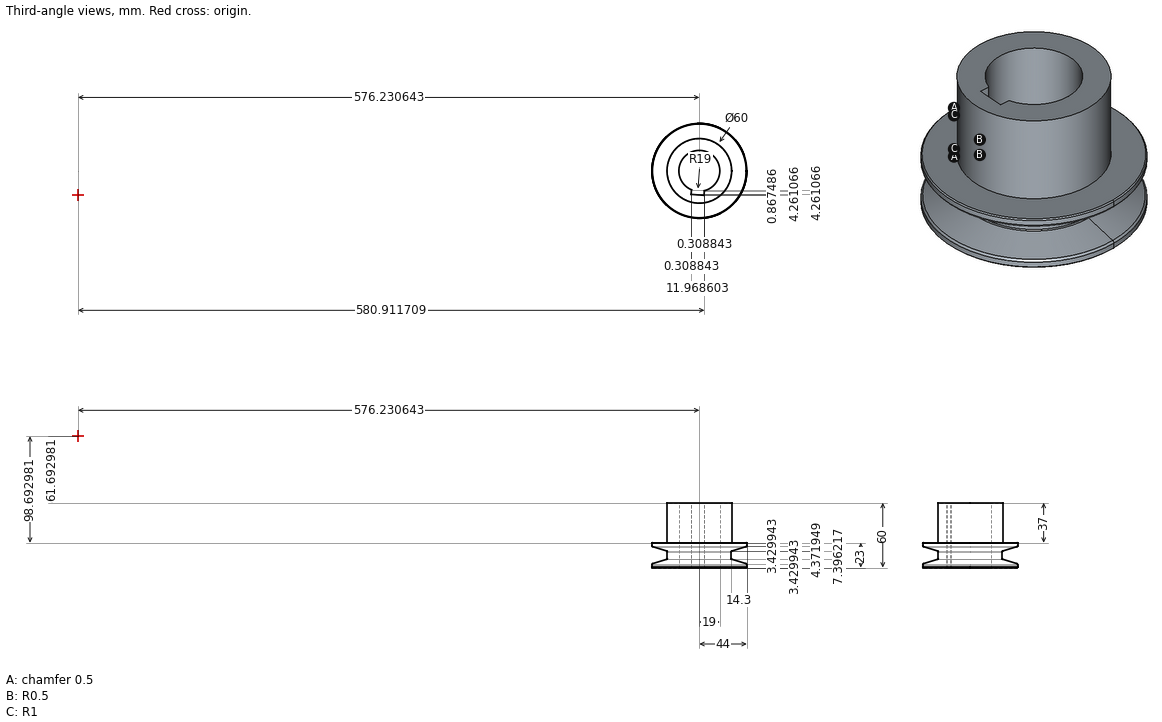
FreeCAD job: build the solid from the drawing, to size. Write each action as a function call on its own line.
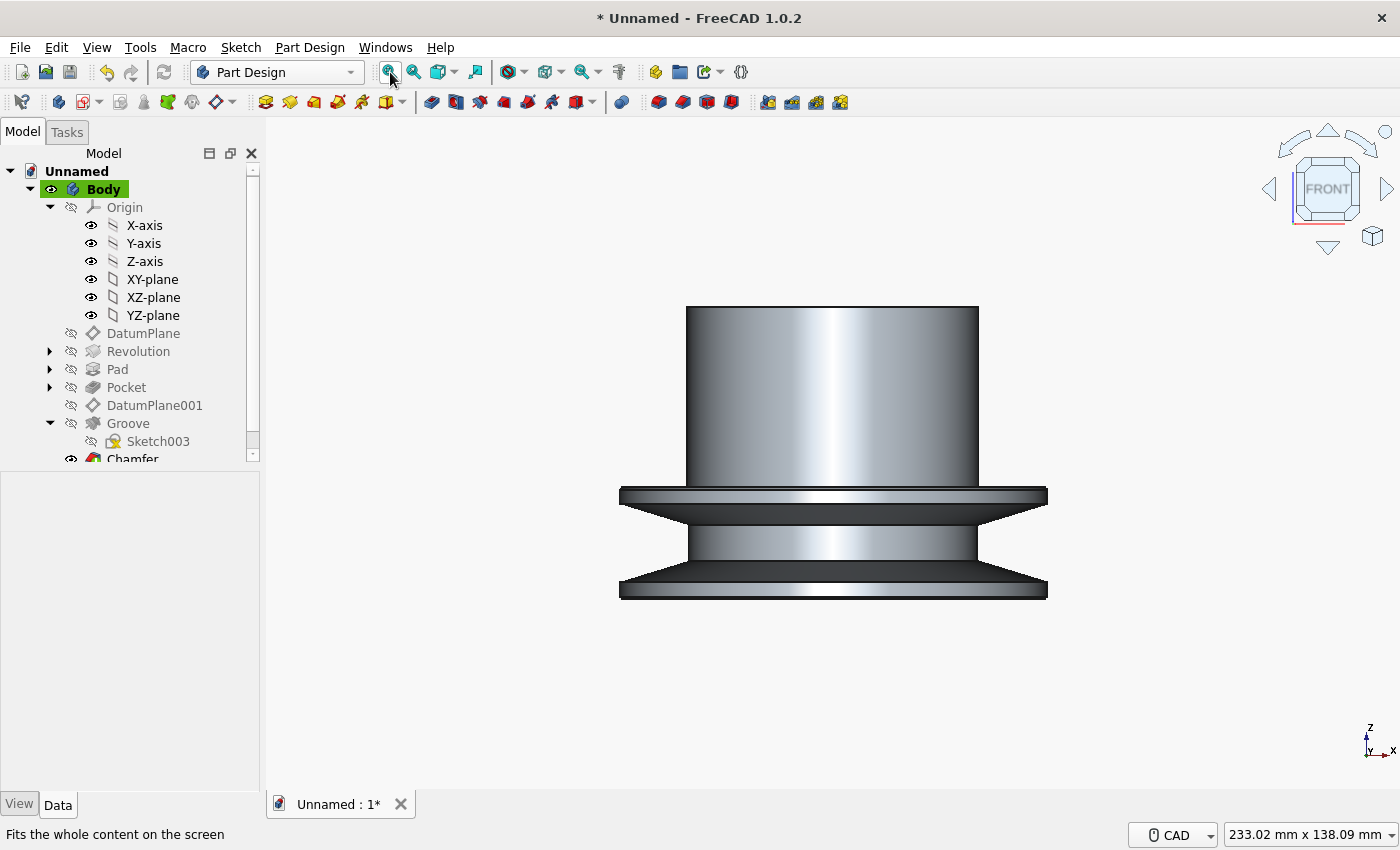
key(3)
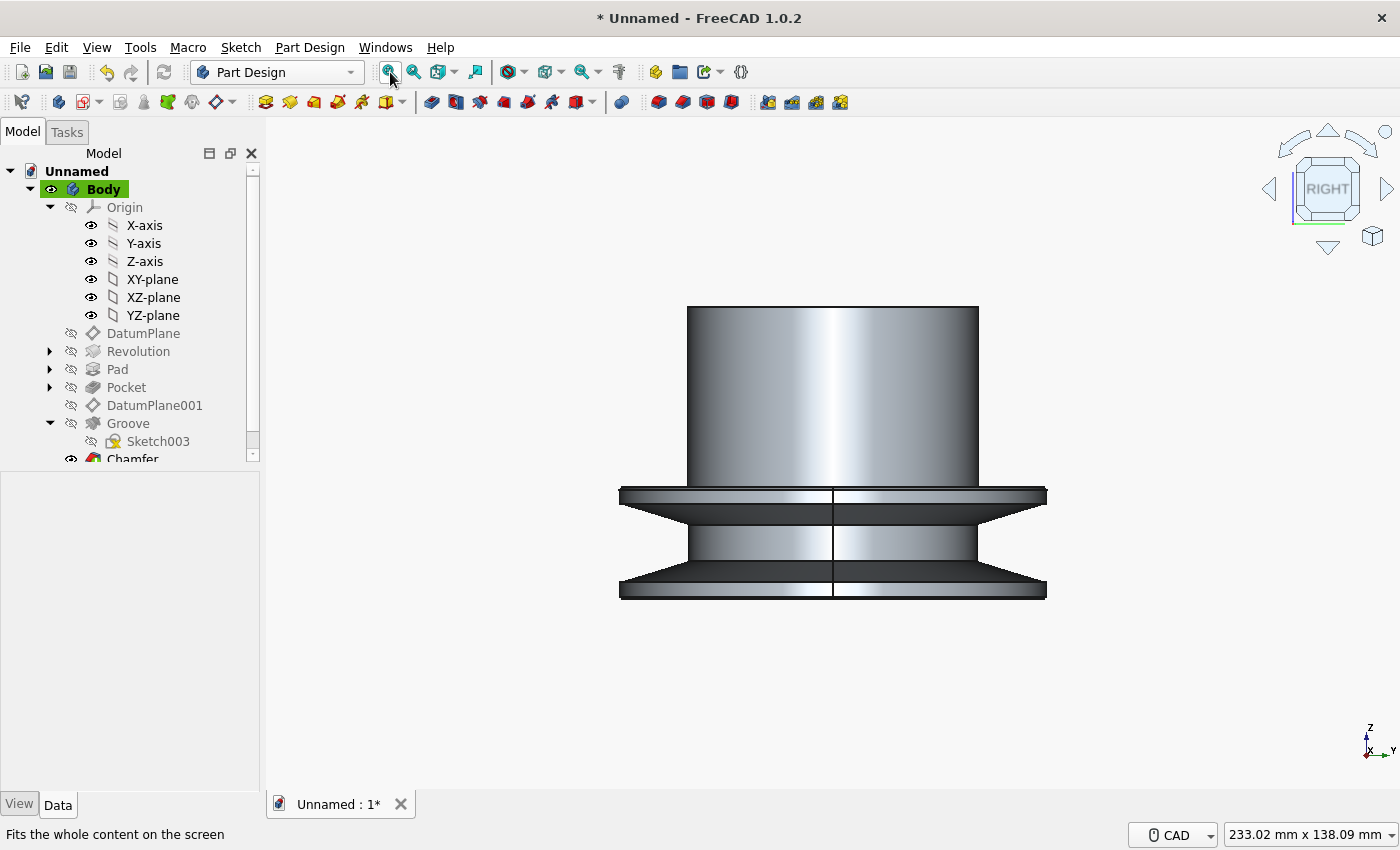
key(v)
key(f)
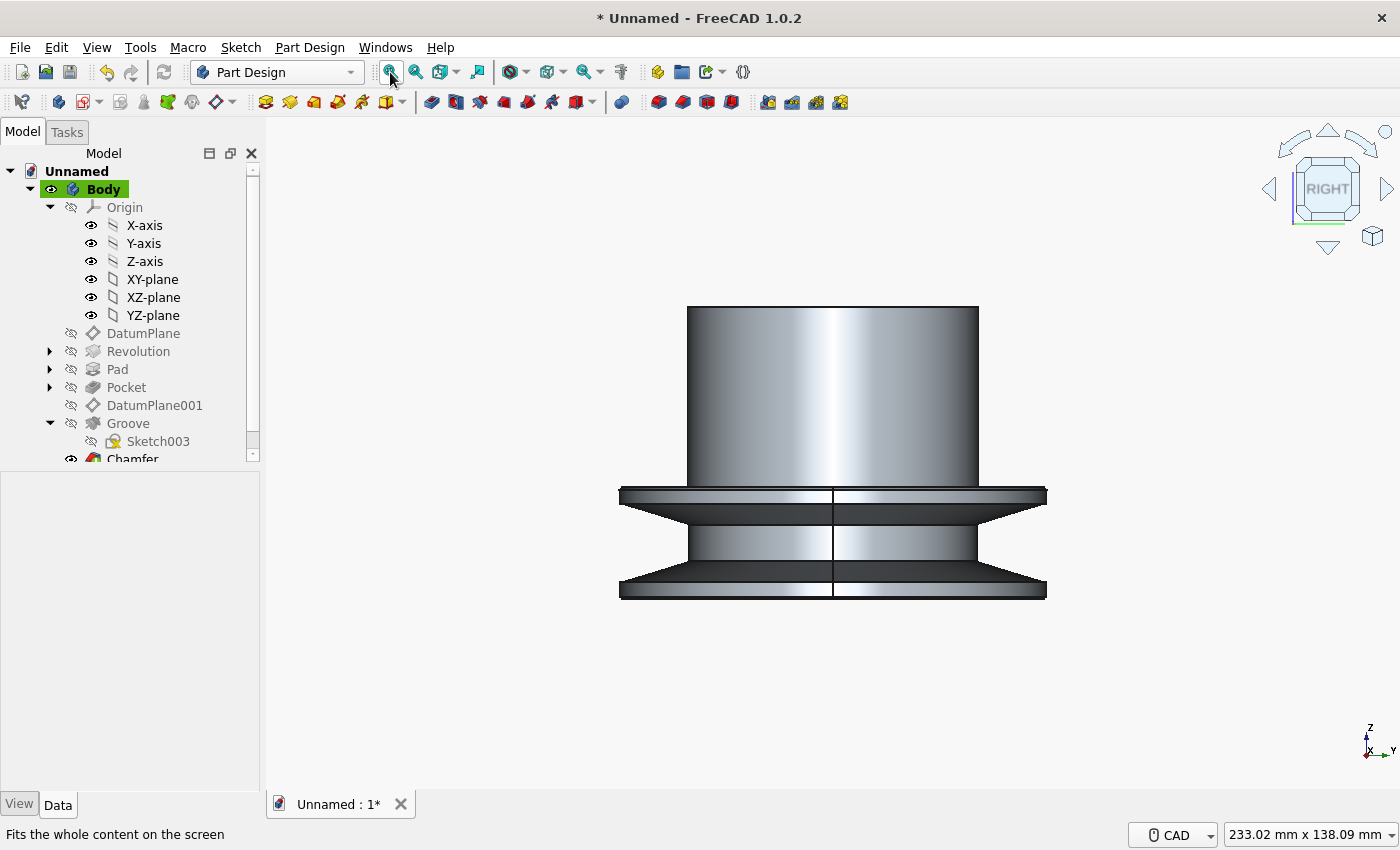
key(5)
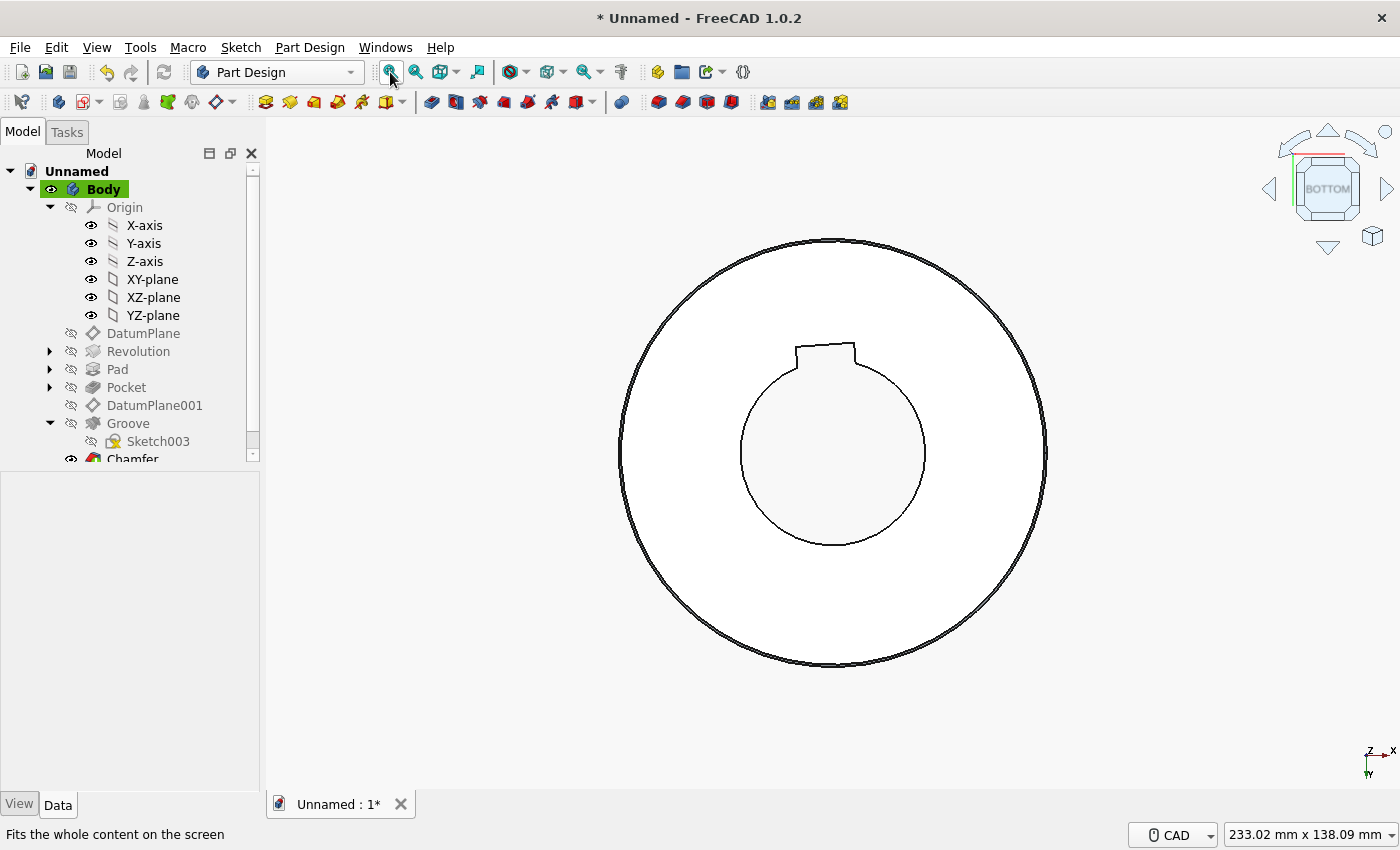
key(4)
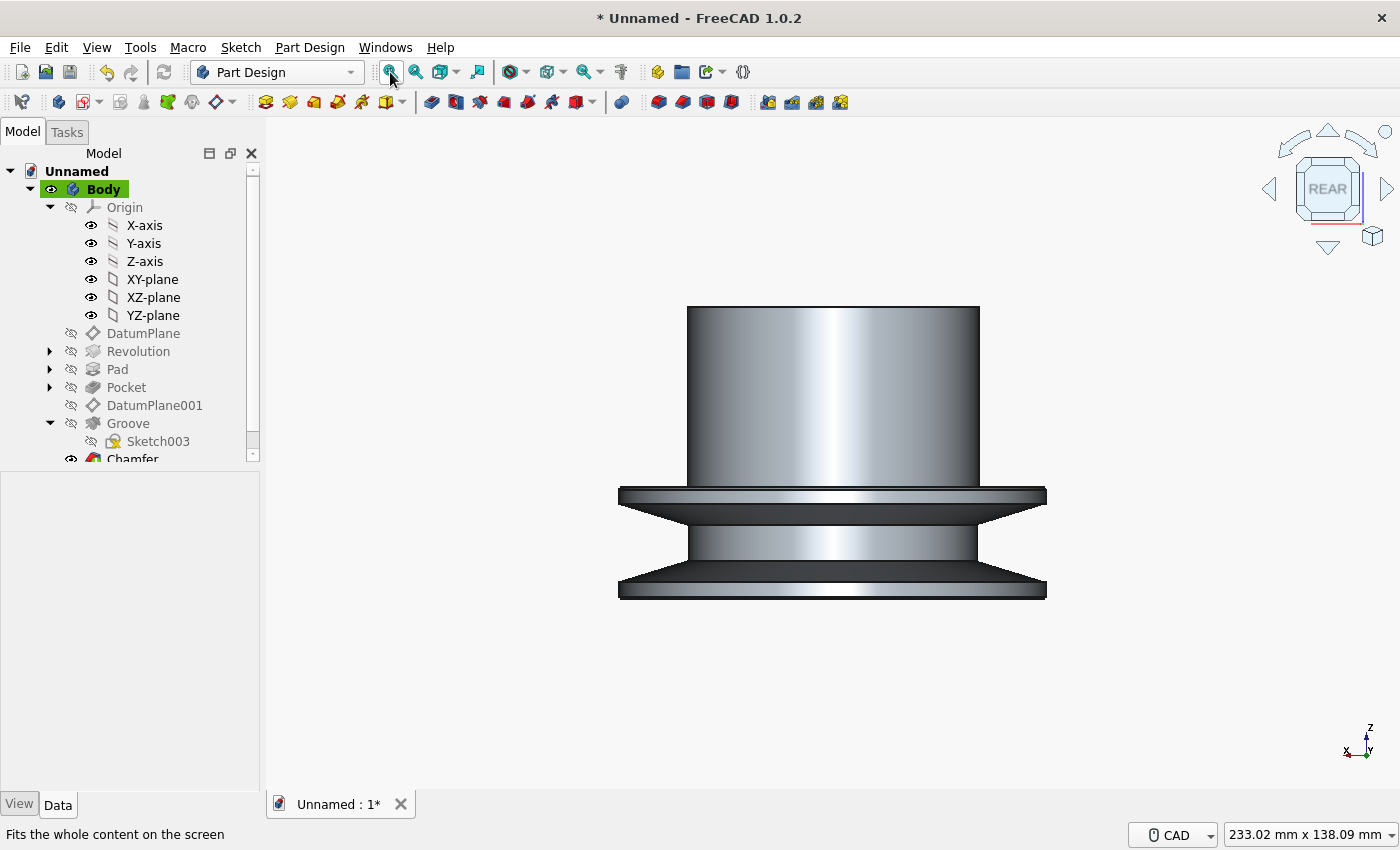
click(392, 72)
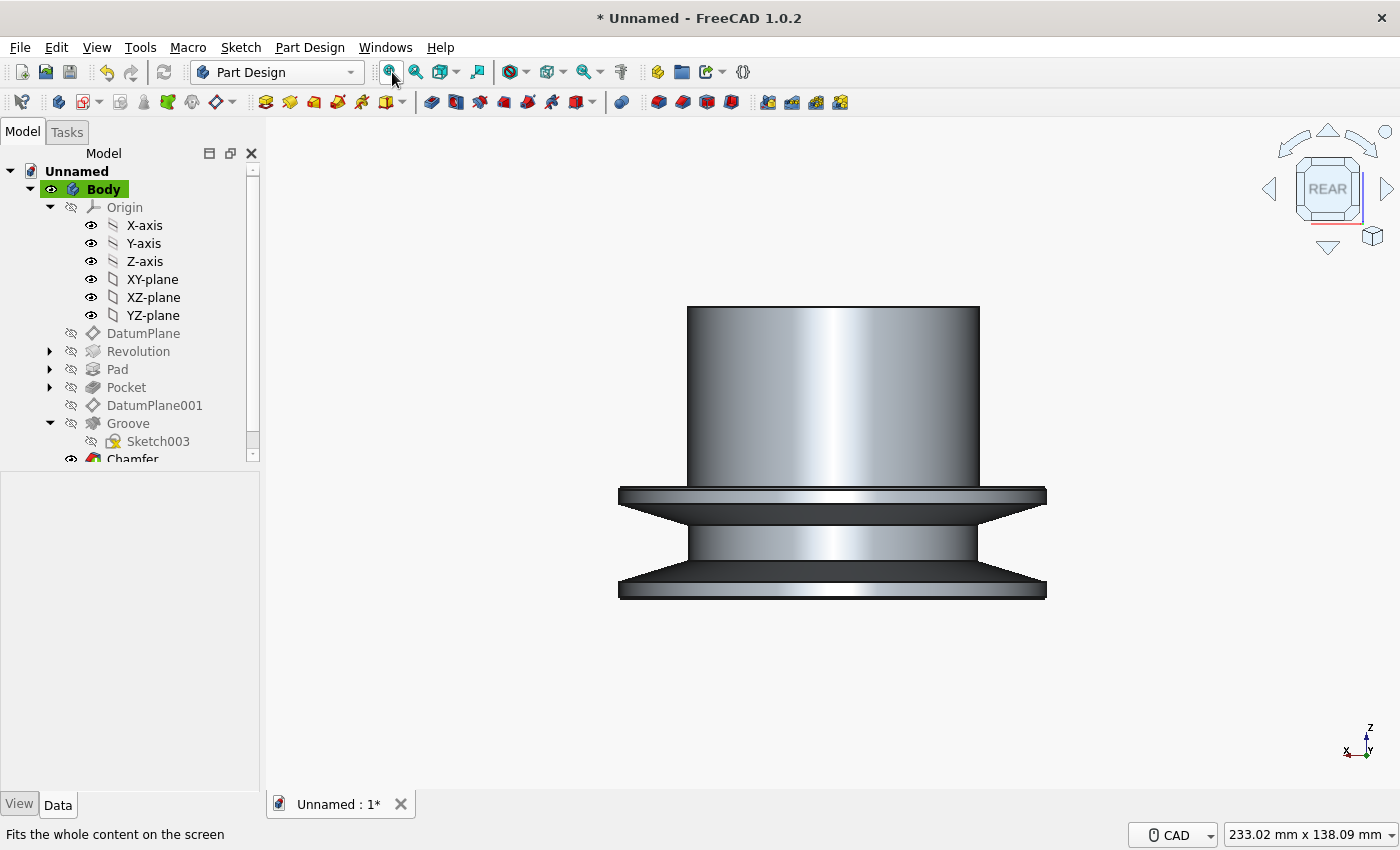
key(6)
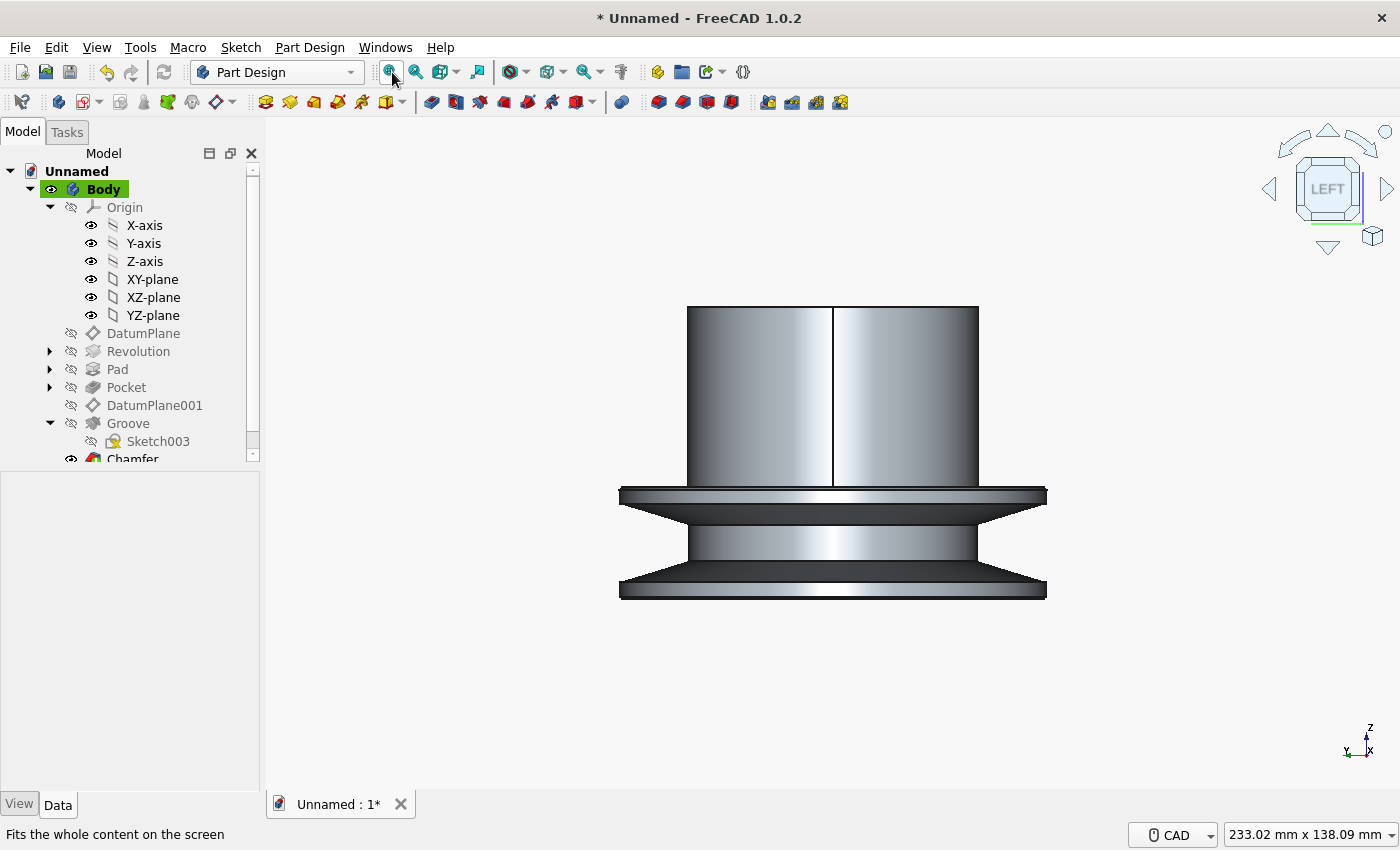
click(392, 72)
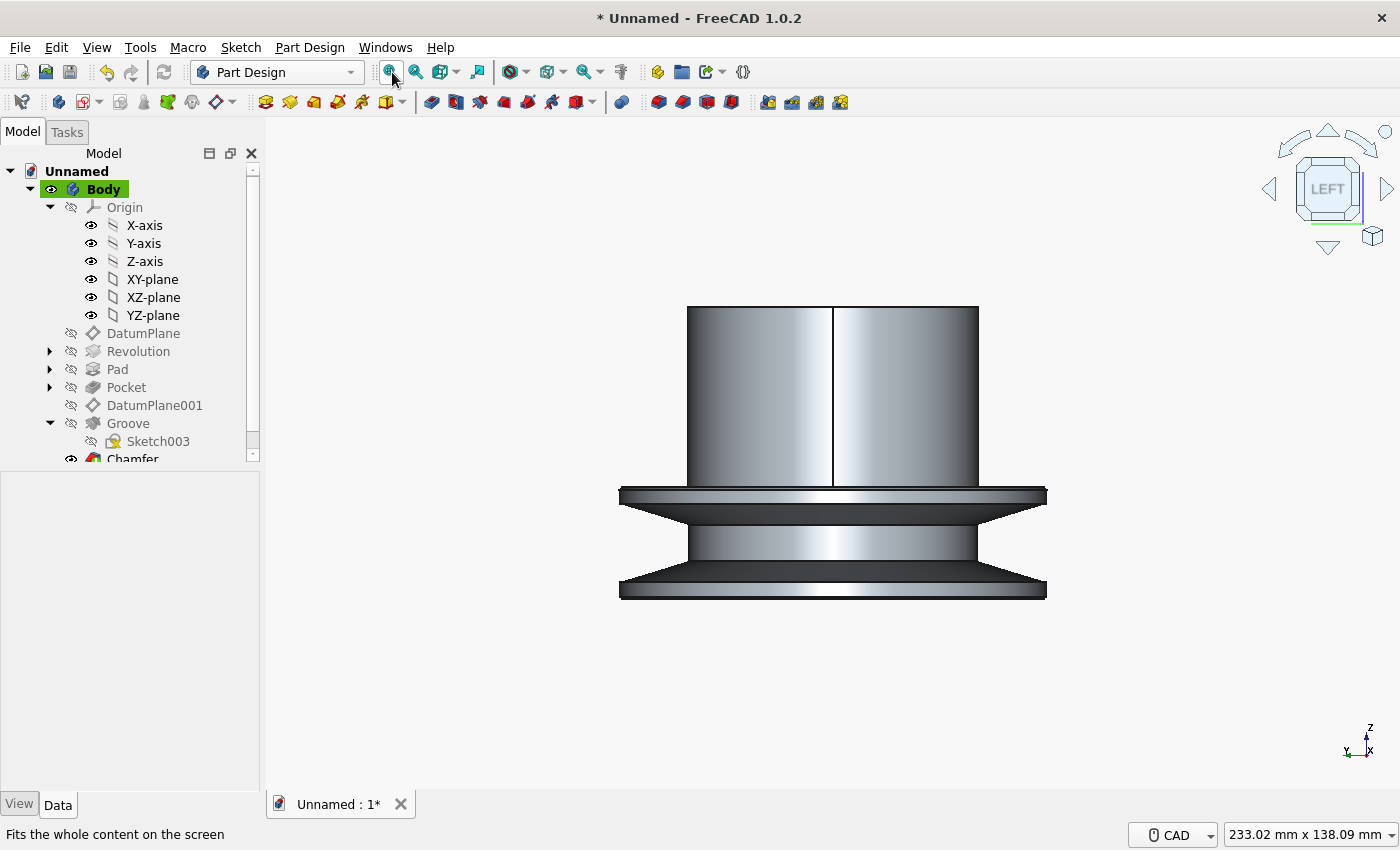
key(v)
key(3)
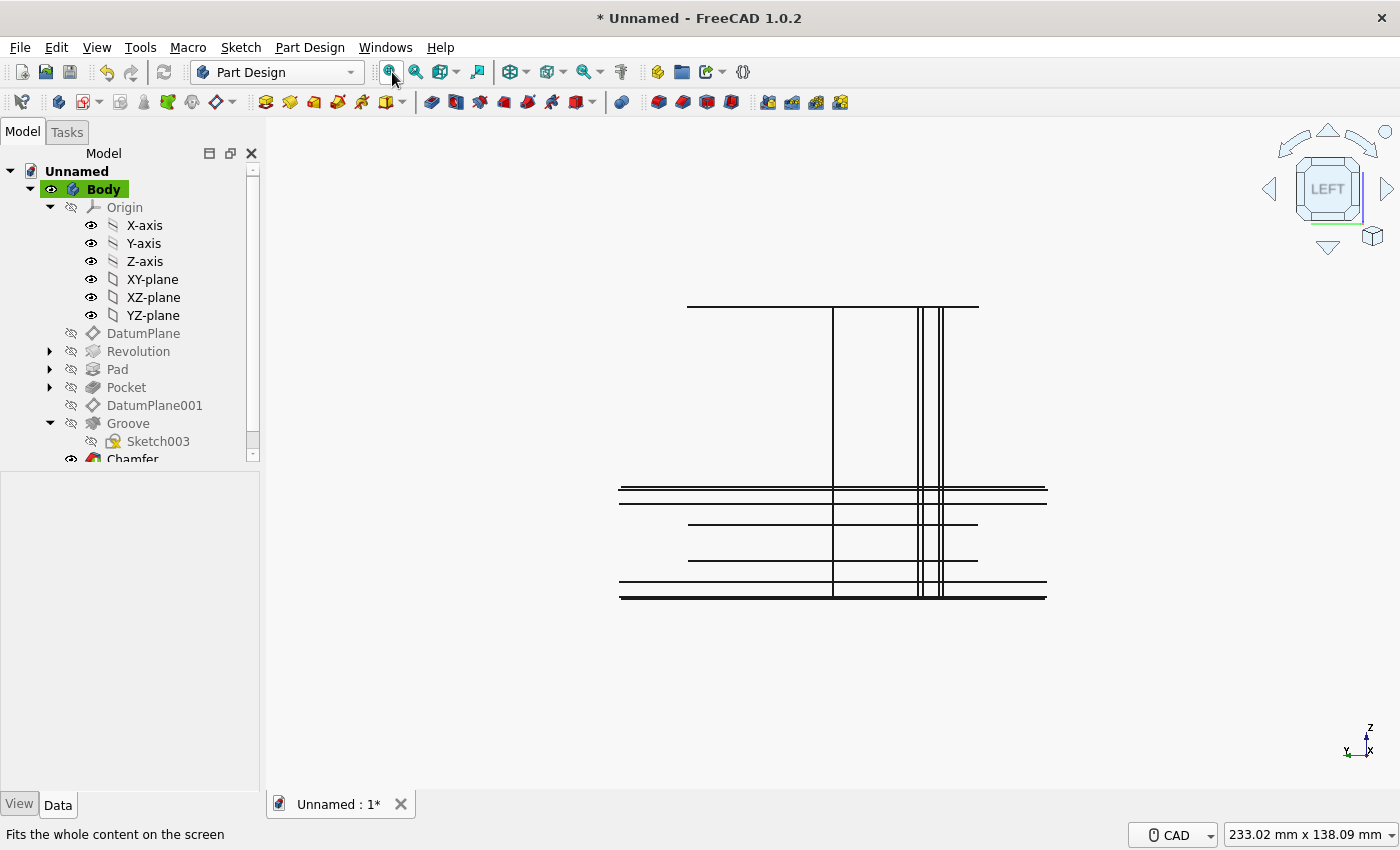
key(0)